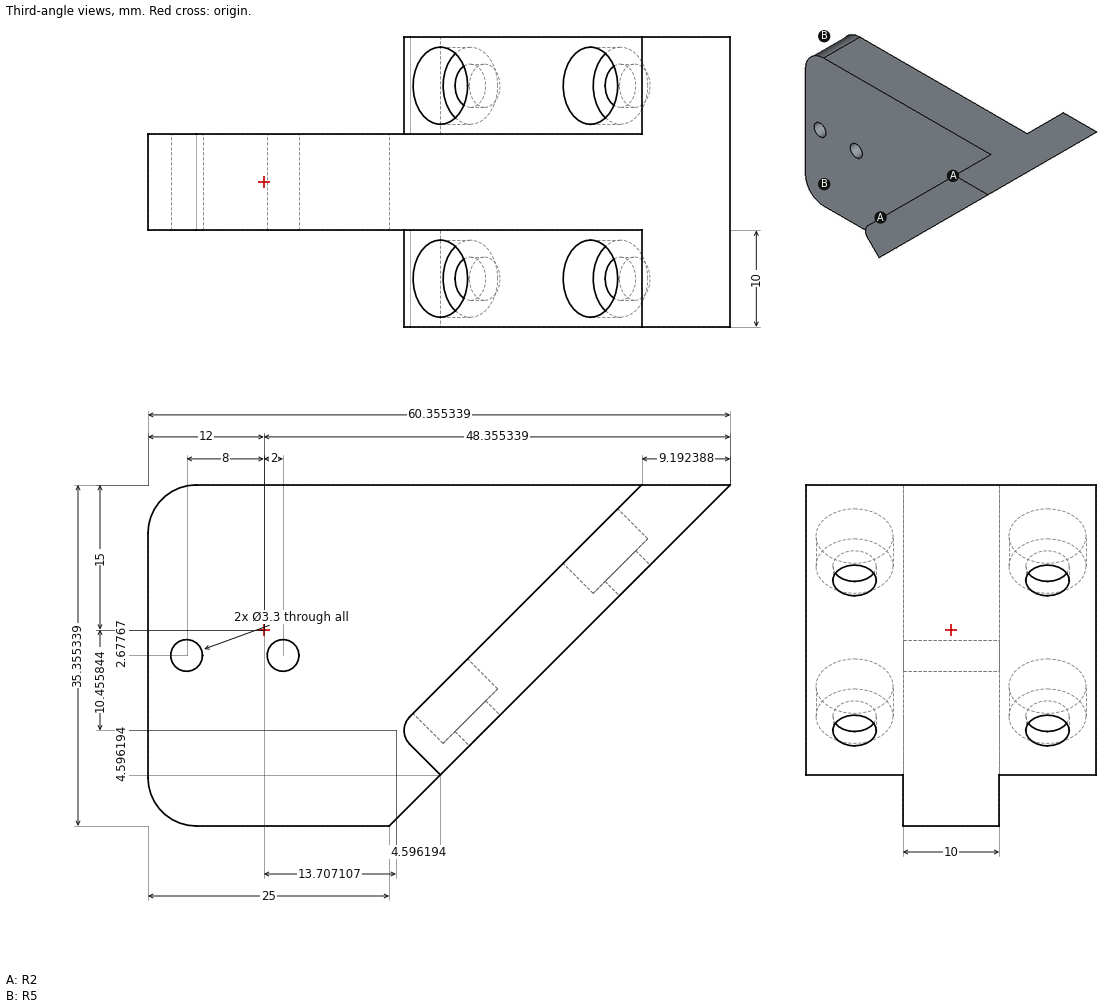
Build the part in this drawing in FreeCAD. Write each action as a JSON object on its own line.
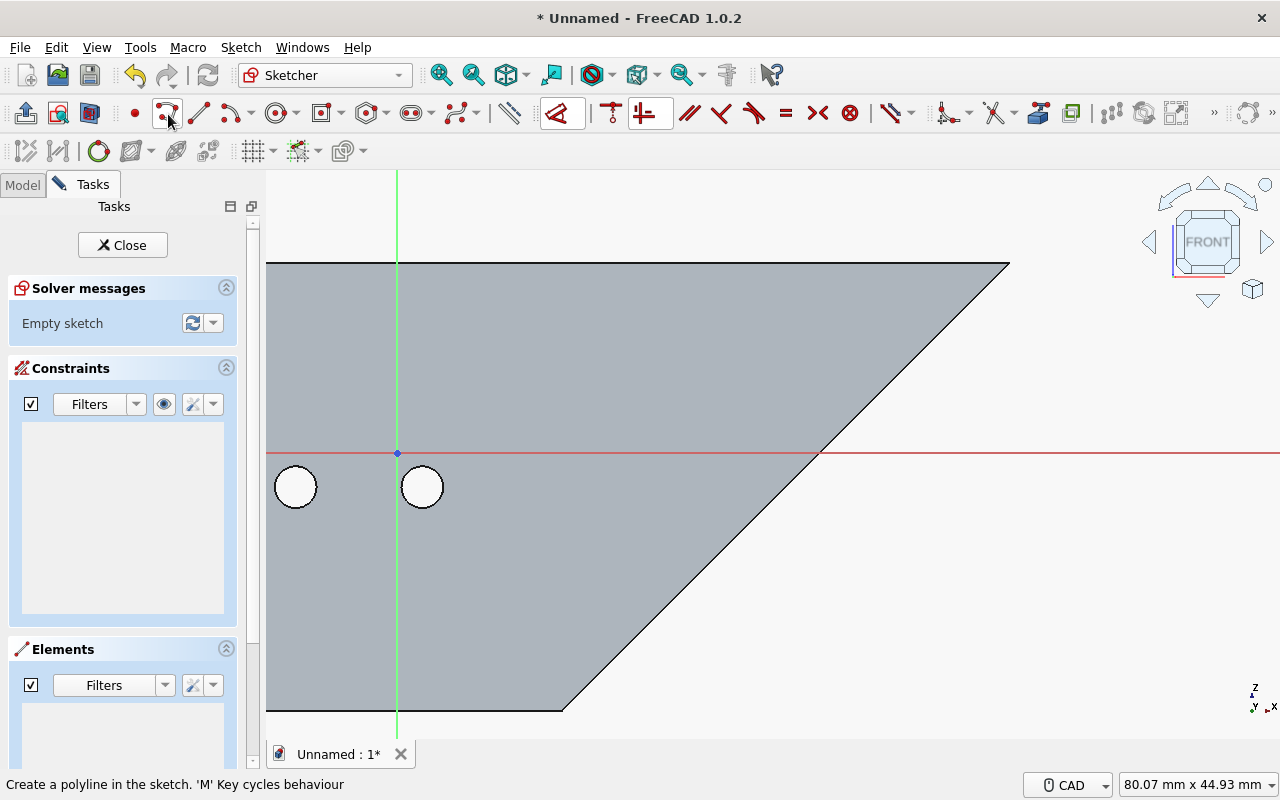
{"action": "left_click", "coordinate": [571, 586]}
{"action": "left_click", "coordinate": [629, 644]}
{"action": "left_click", "coordinate": [1009, 263]}
{"action": "left_click", "coordinate": [893, 263]}
{"action": "left_click", "coordinate": [571, 587]}
{"action": "key", "text": "Escape"}
{"action": "key", "text": "Escape"}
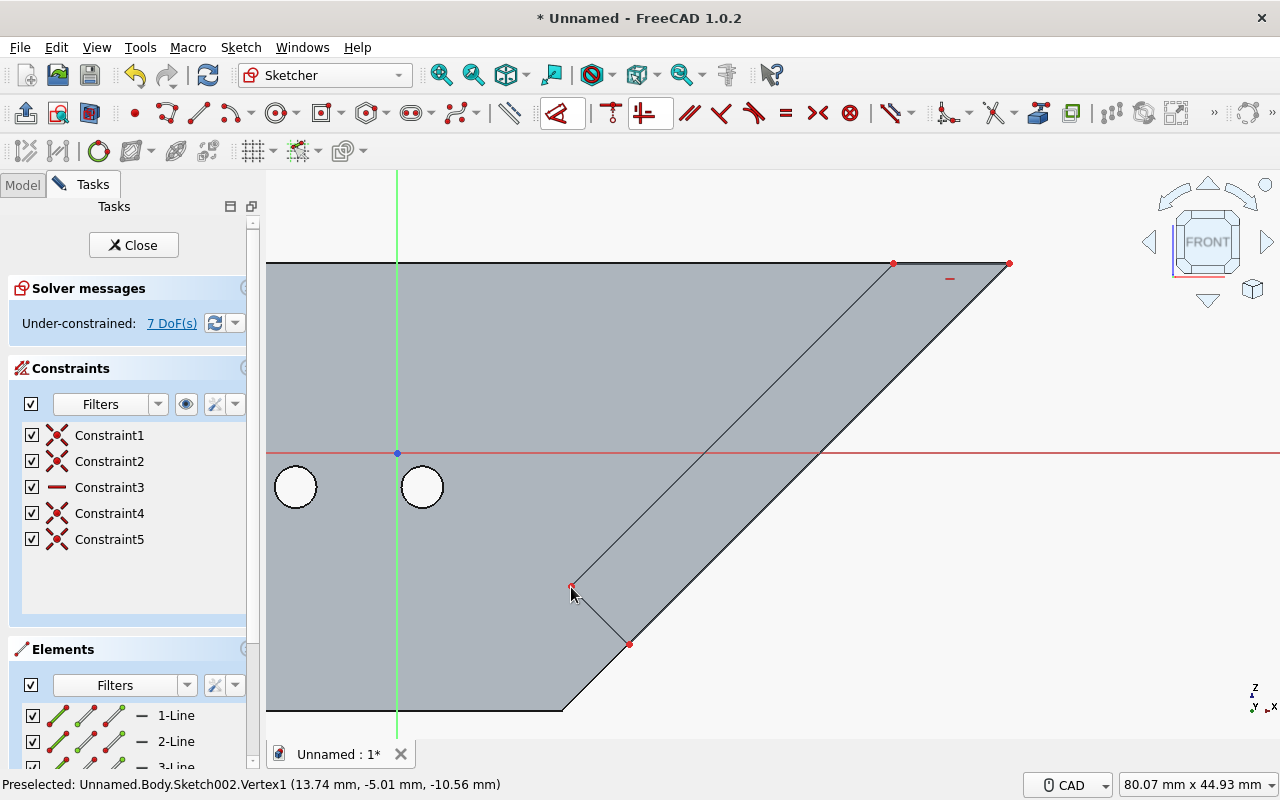
{"action": "left_click", "coordinate": [1009, 264]}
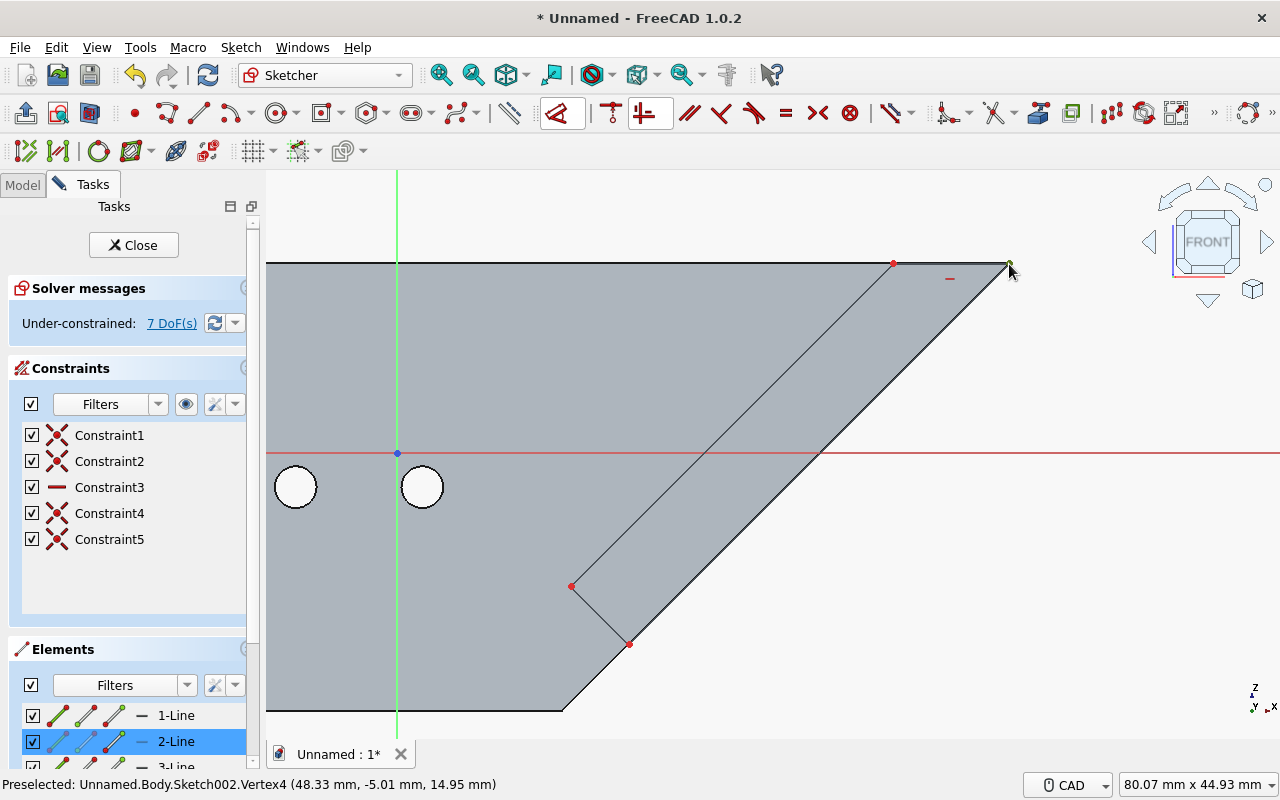
{"action": "left_click", "coordinate": [580, 114]}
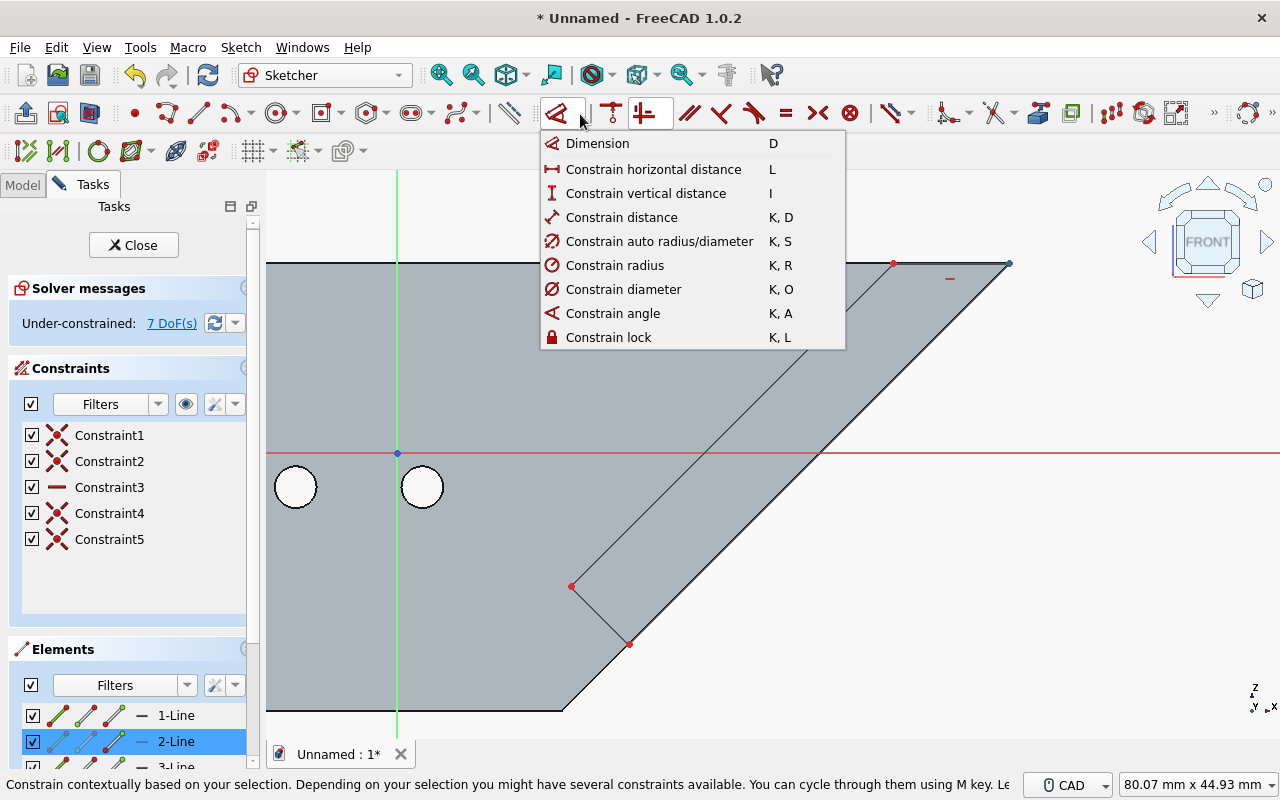
{"action": "left_click", "coordinate": [693, 193]}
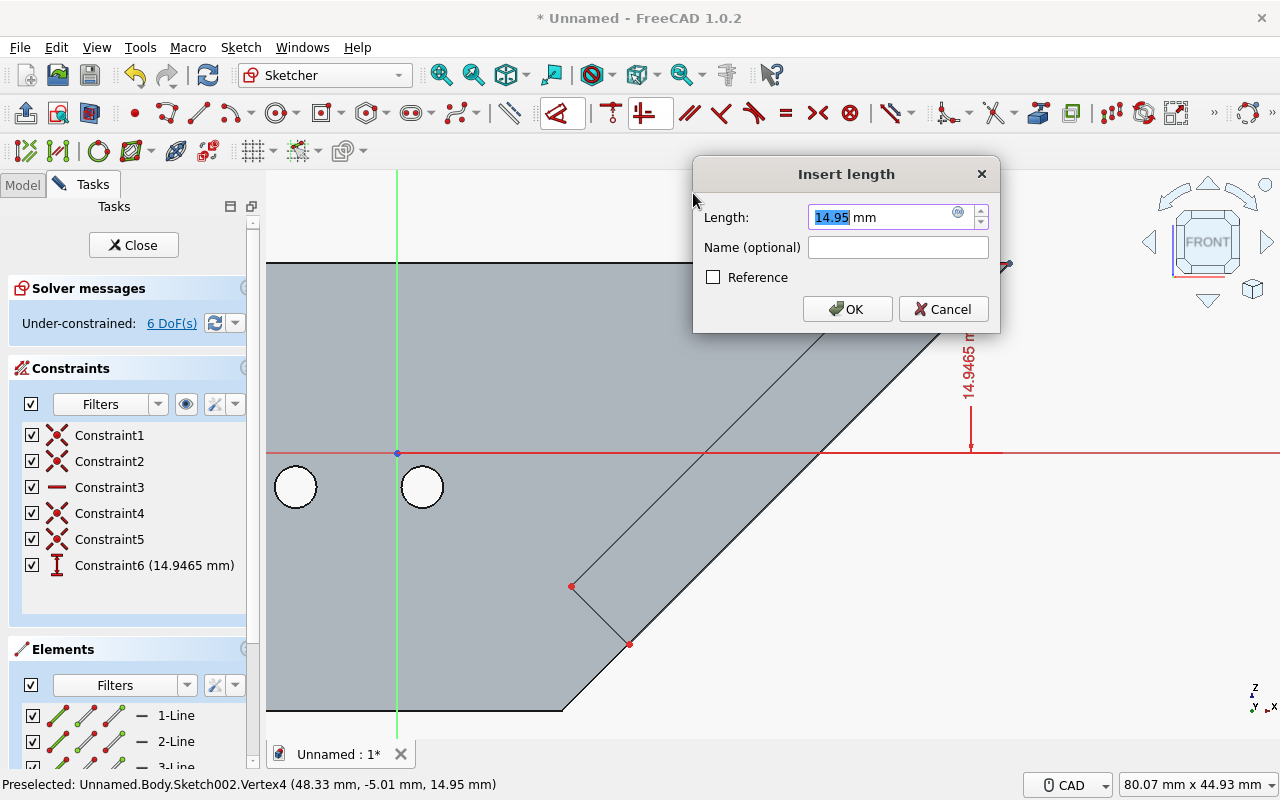
{"action": "type", "text": "15"}
{"action": "key", "text": "Return"}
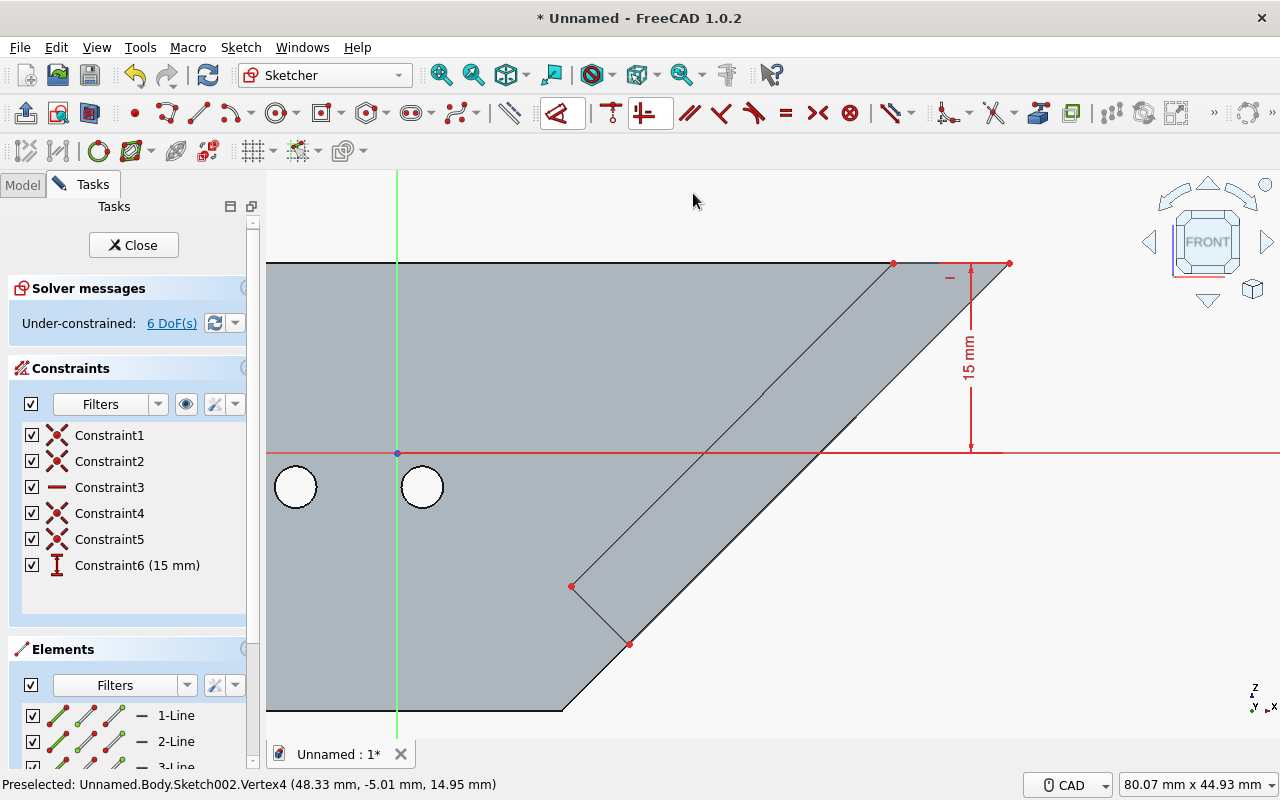
{"action": "left_click", "coordinate": [974, 263]}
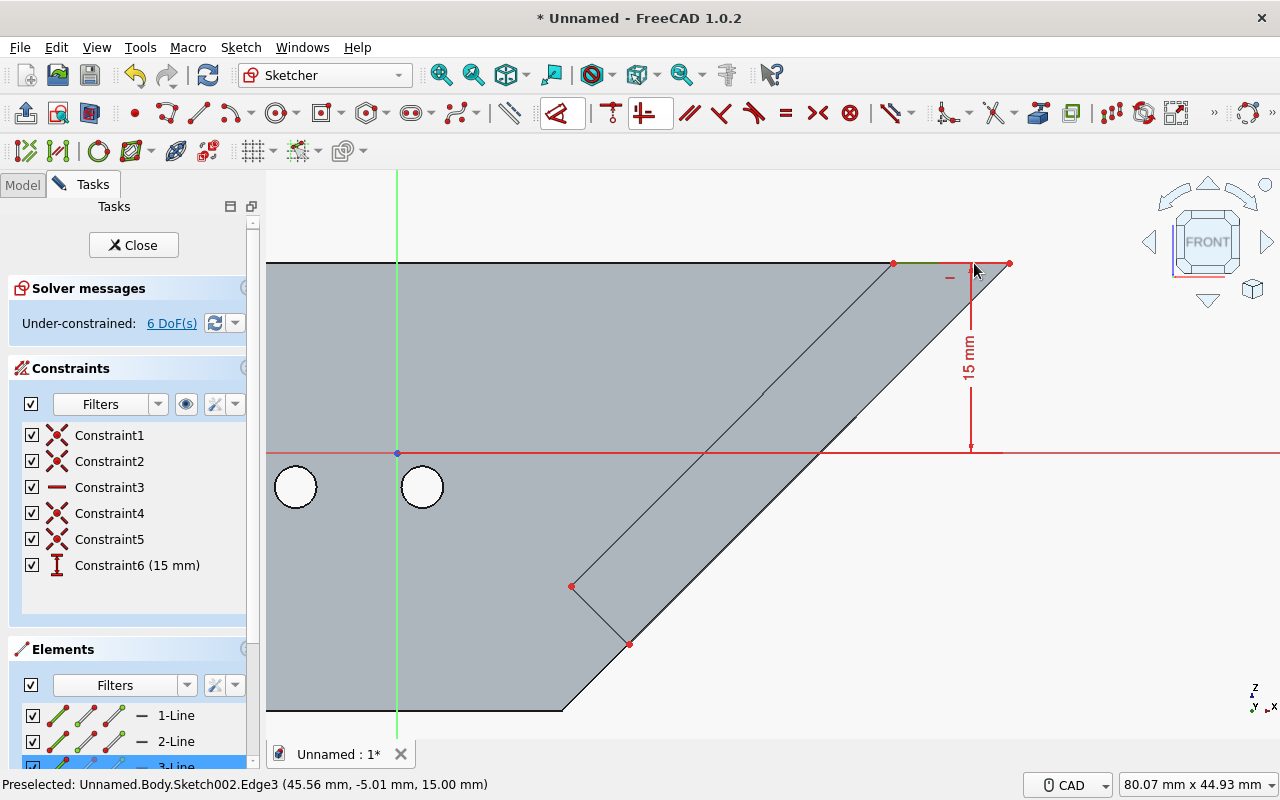
{"action": "left_click", "coordinate": [580, 114]}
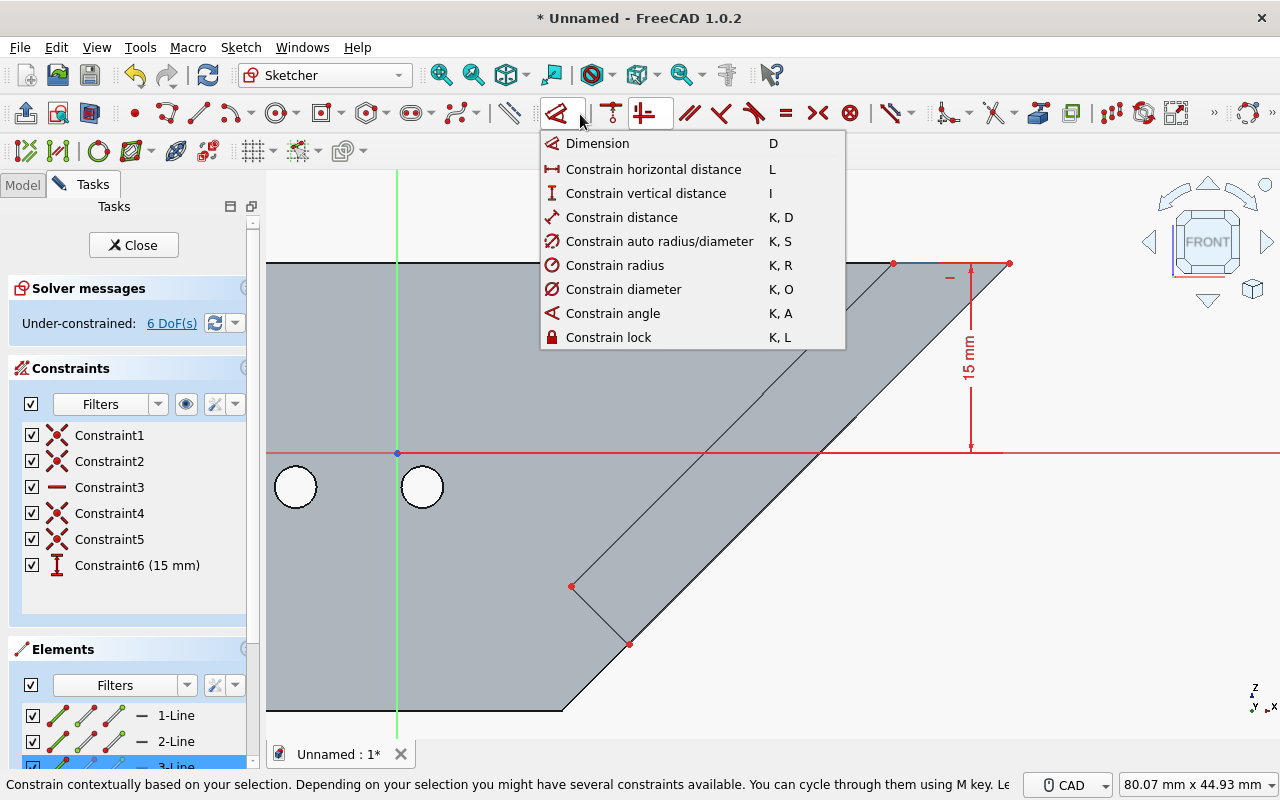
{"action": "left_click", "coordinate": [693, 169]}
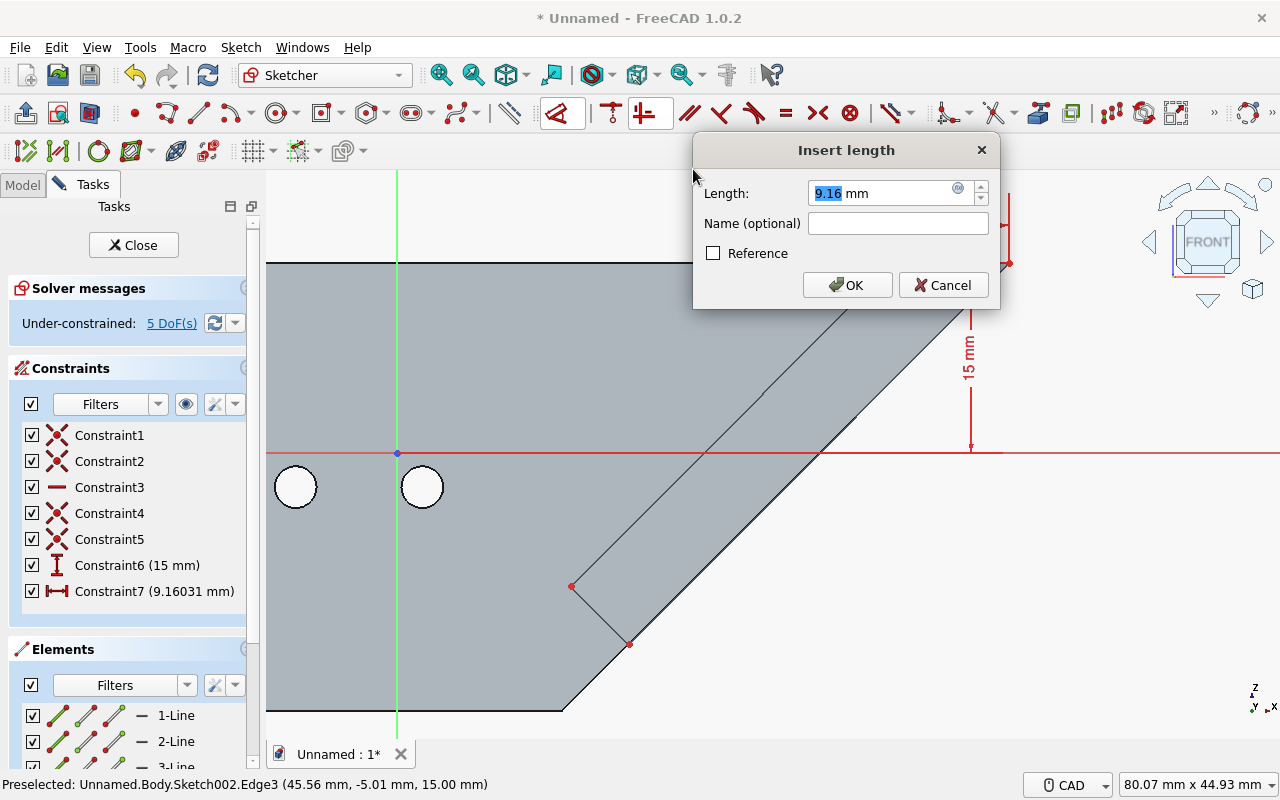
{"action": "type", "text": "9.192388"}
{"action": "key", "text": "Return"}